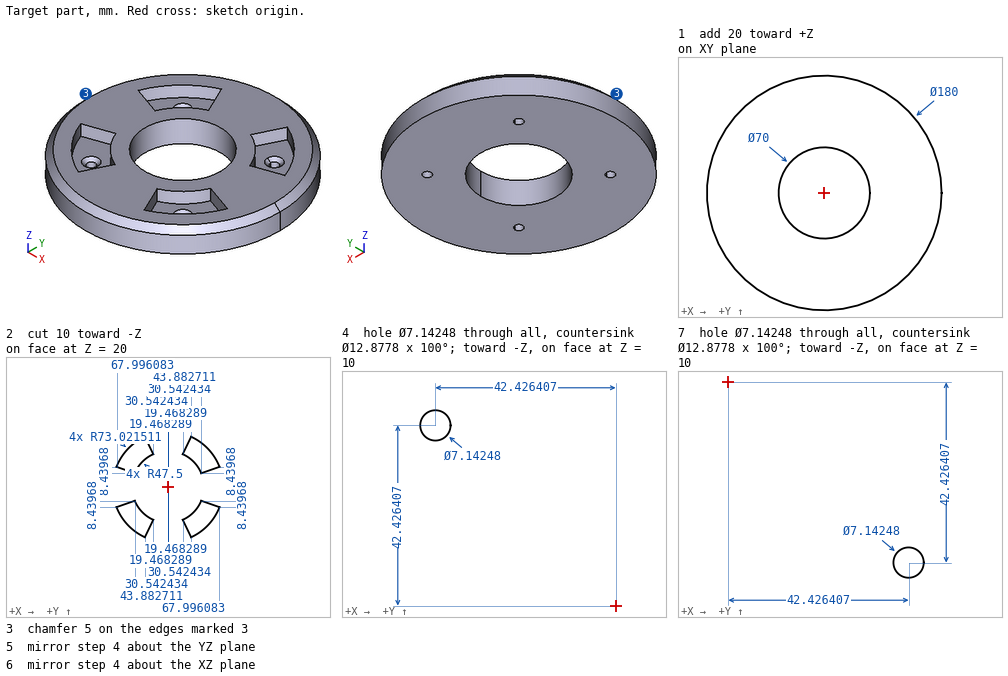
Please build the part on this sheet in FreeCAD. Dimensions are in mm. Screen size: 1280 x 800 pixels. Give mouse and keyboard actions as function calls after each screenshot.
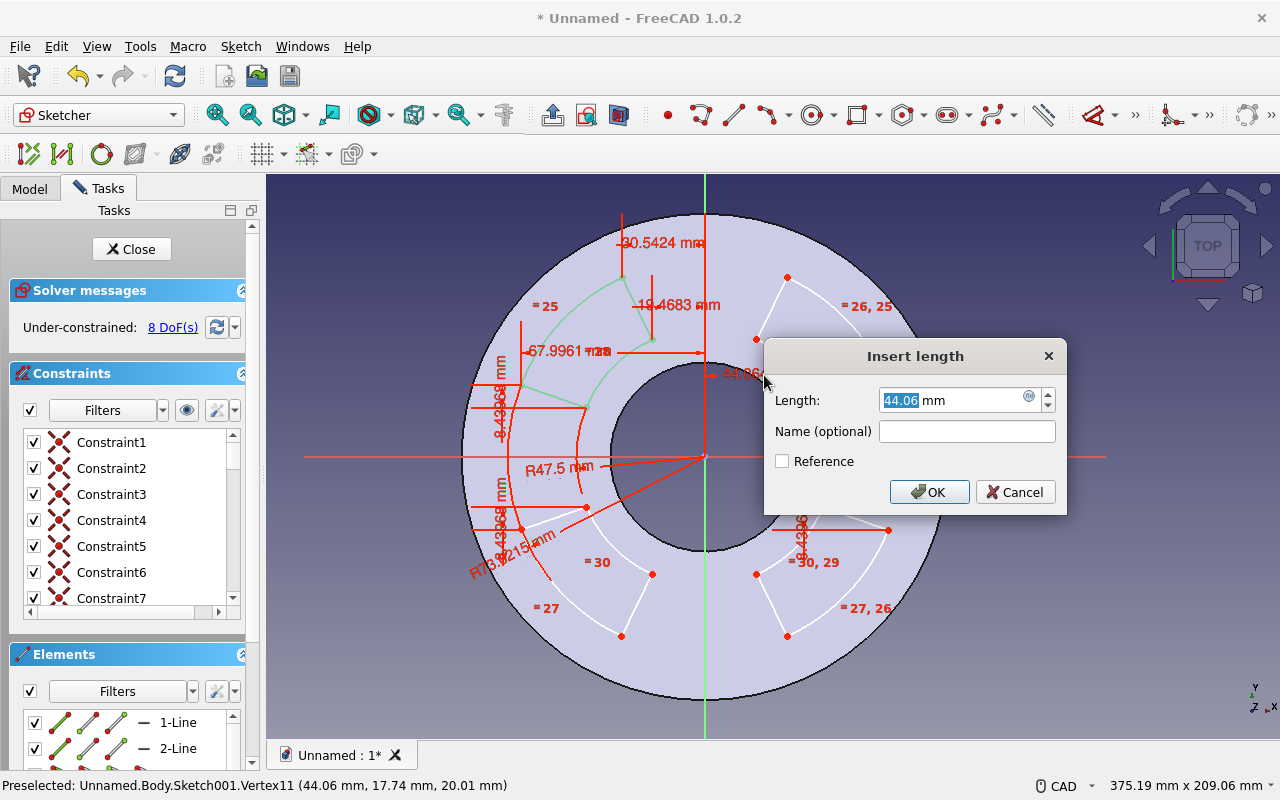
text(43.882711)
key(Return)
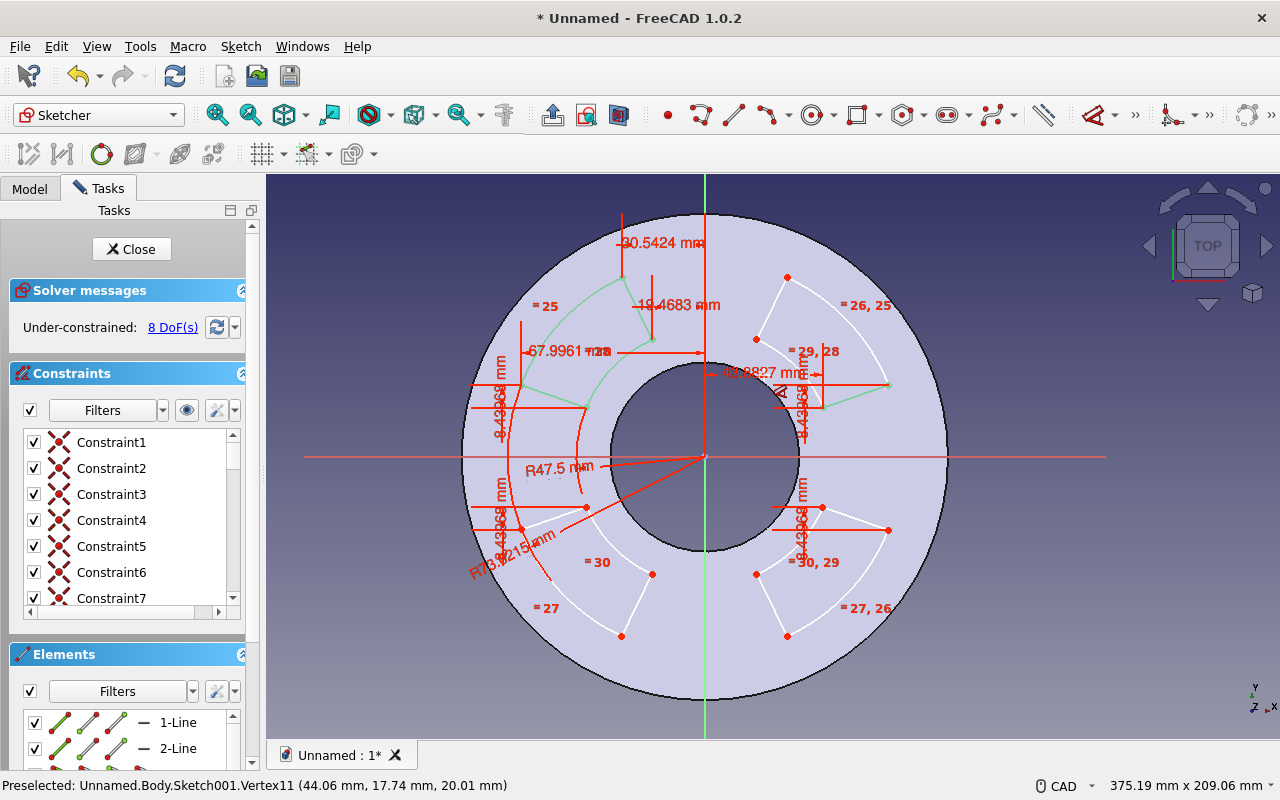
click(787, 278)
click(746, 244)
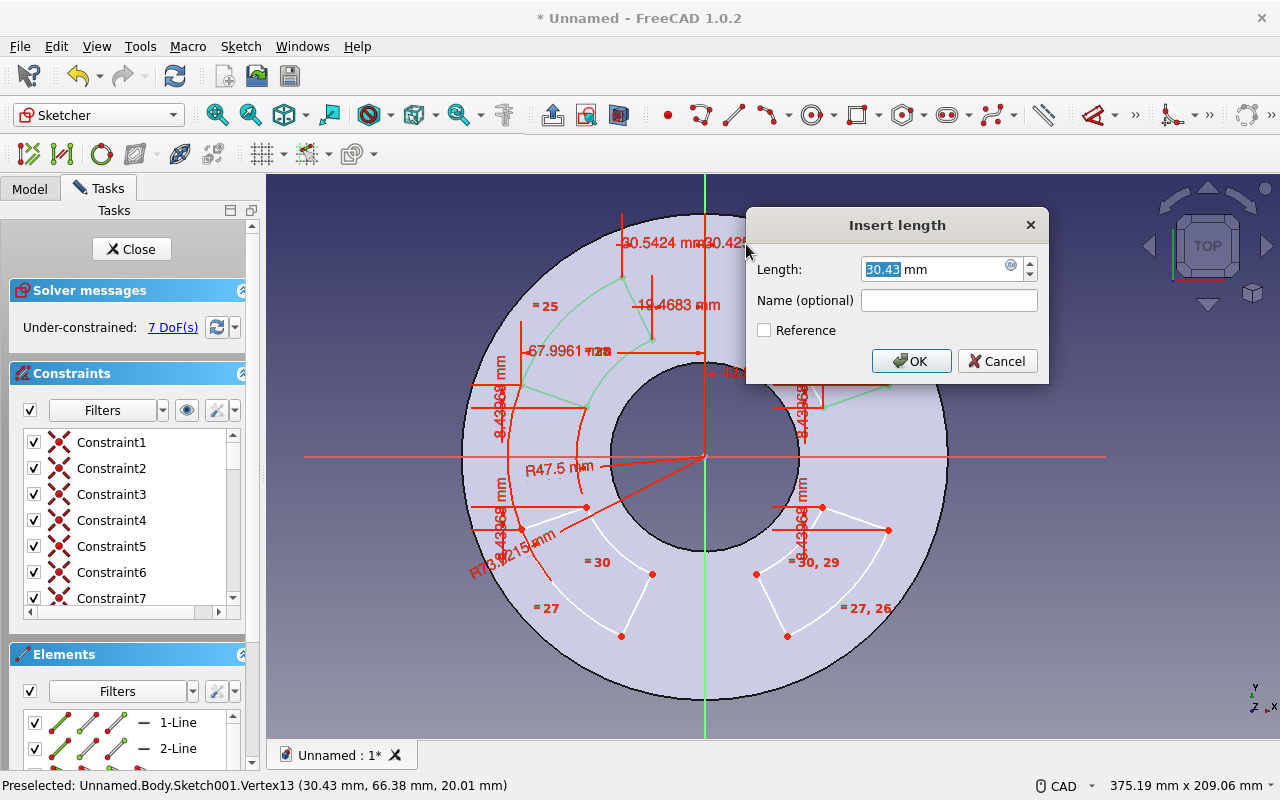
text(30.542434)
key(Return)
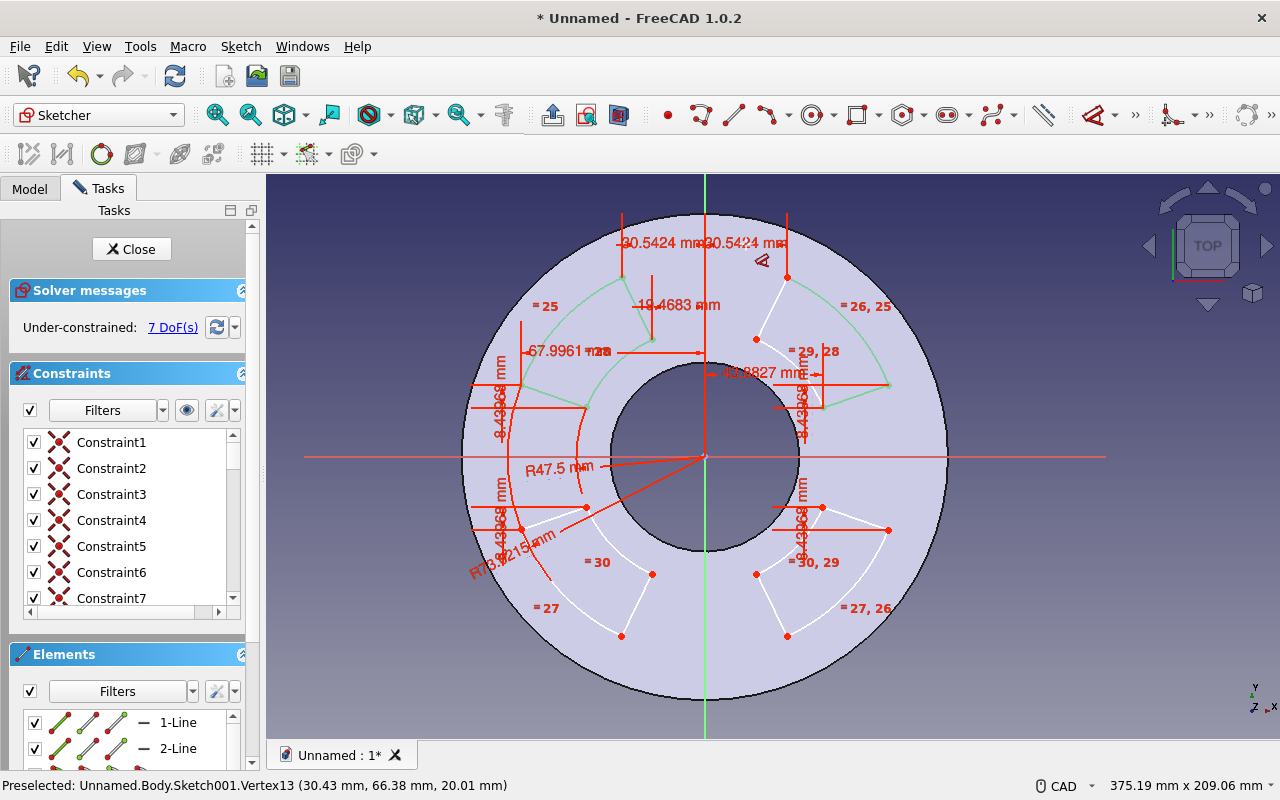
click(757, 340)
click(749, 306)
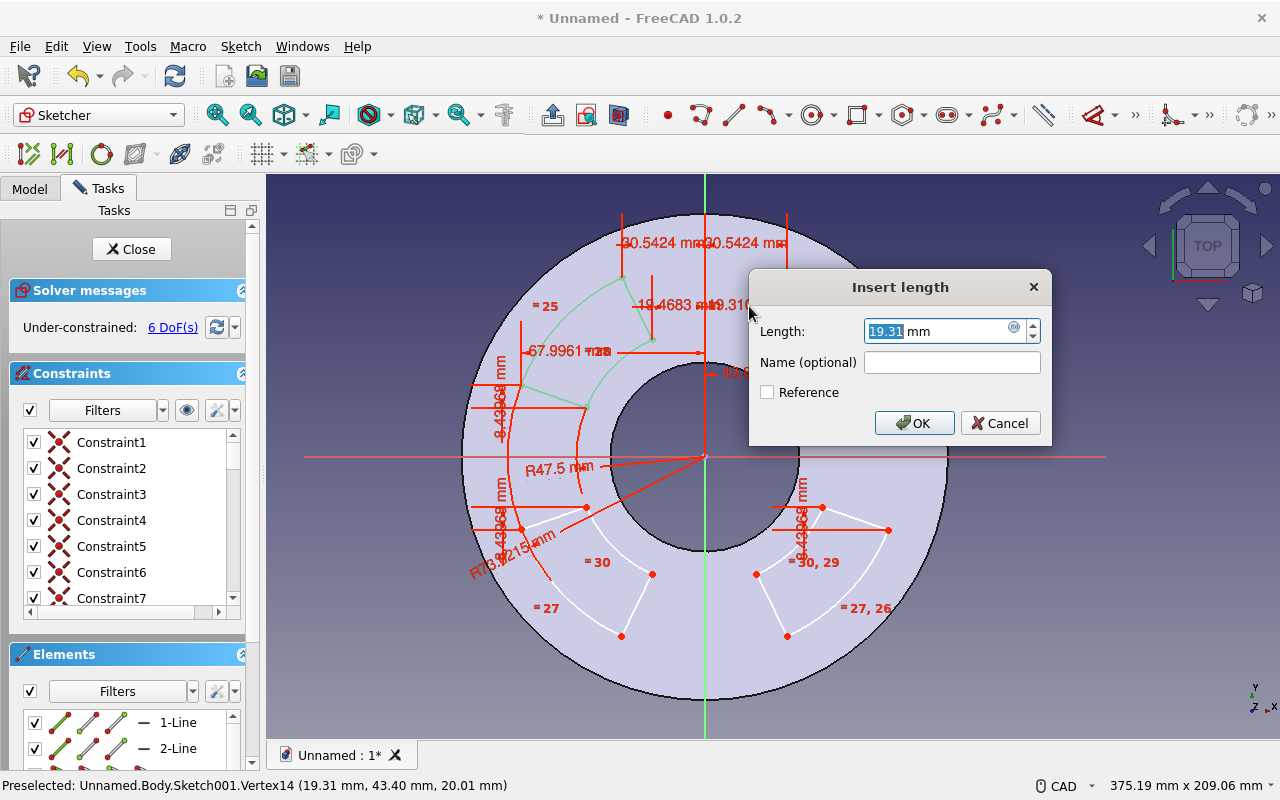
text(19.468289)
key(Return)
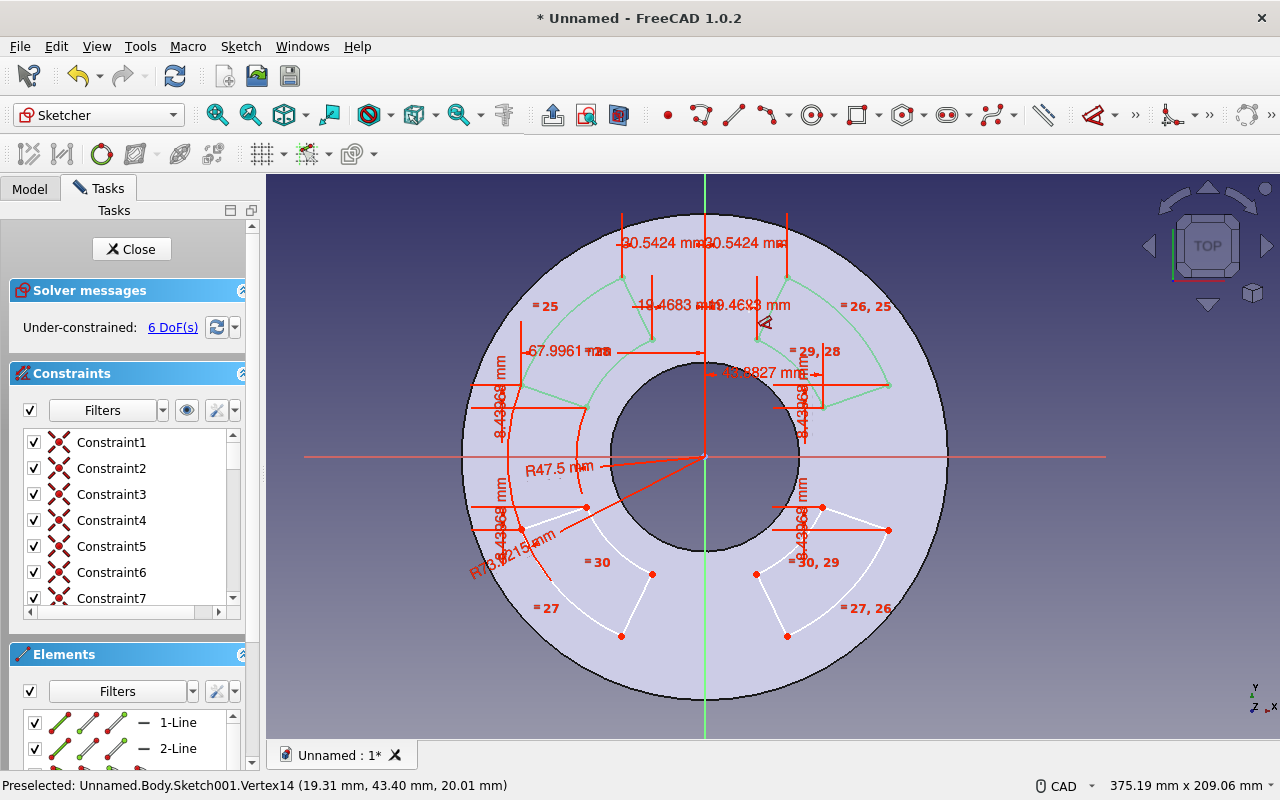
click(757, 574)
click(731, 608)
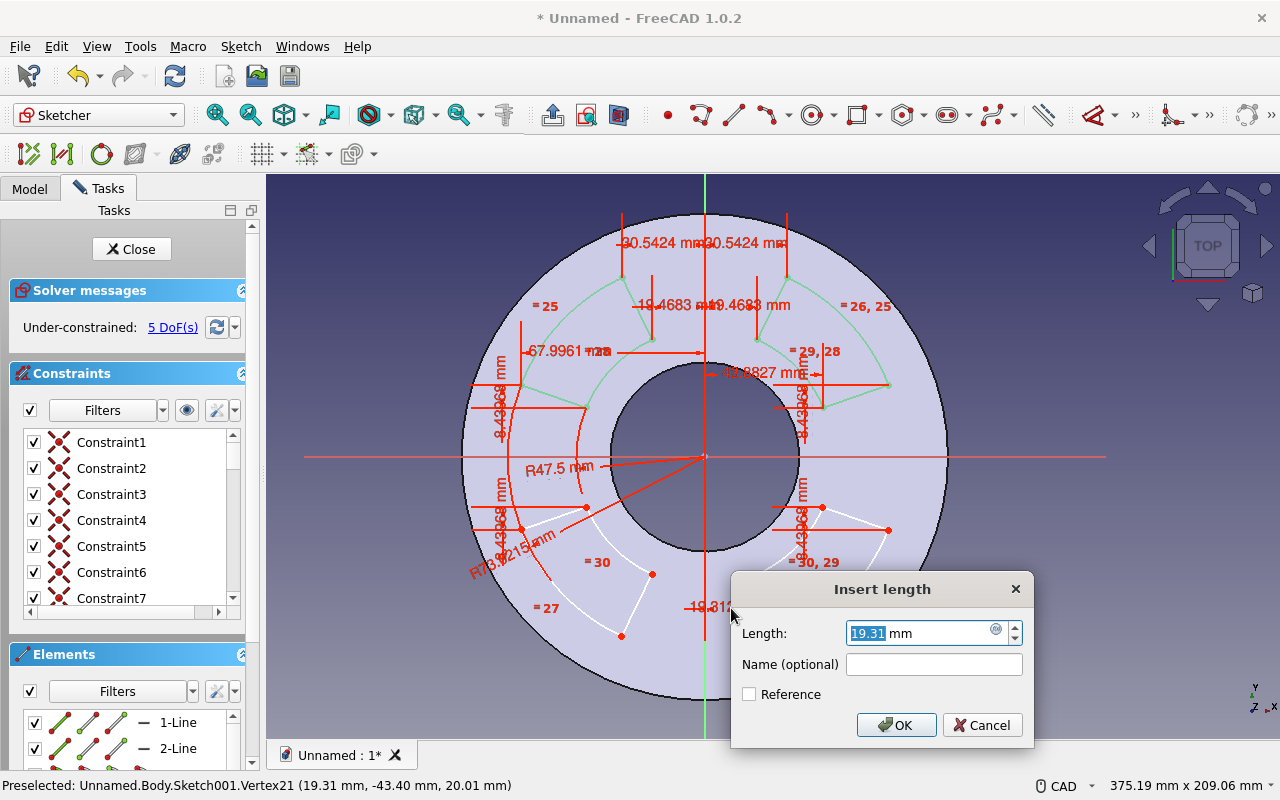
text(19.468289)
key(Return)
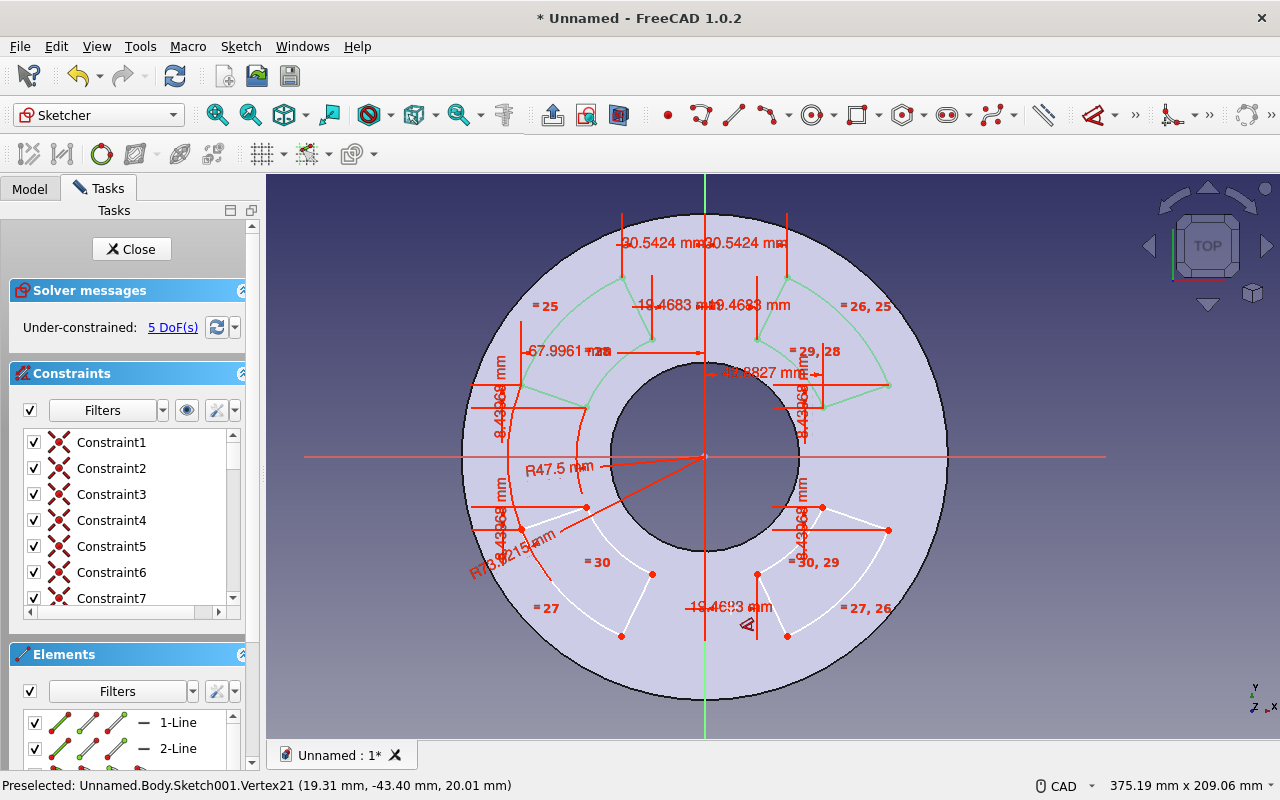
click(787, 636)
click(746, 670)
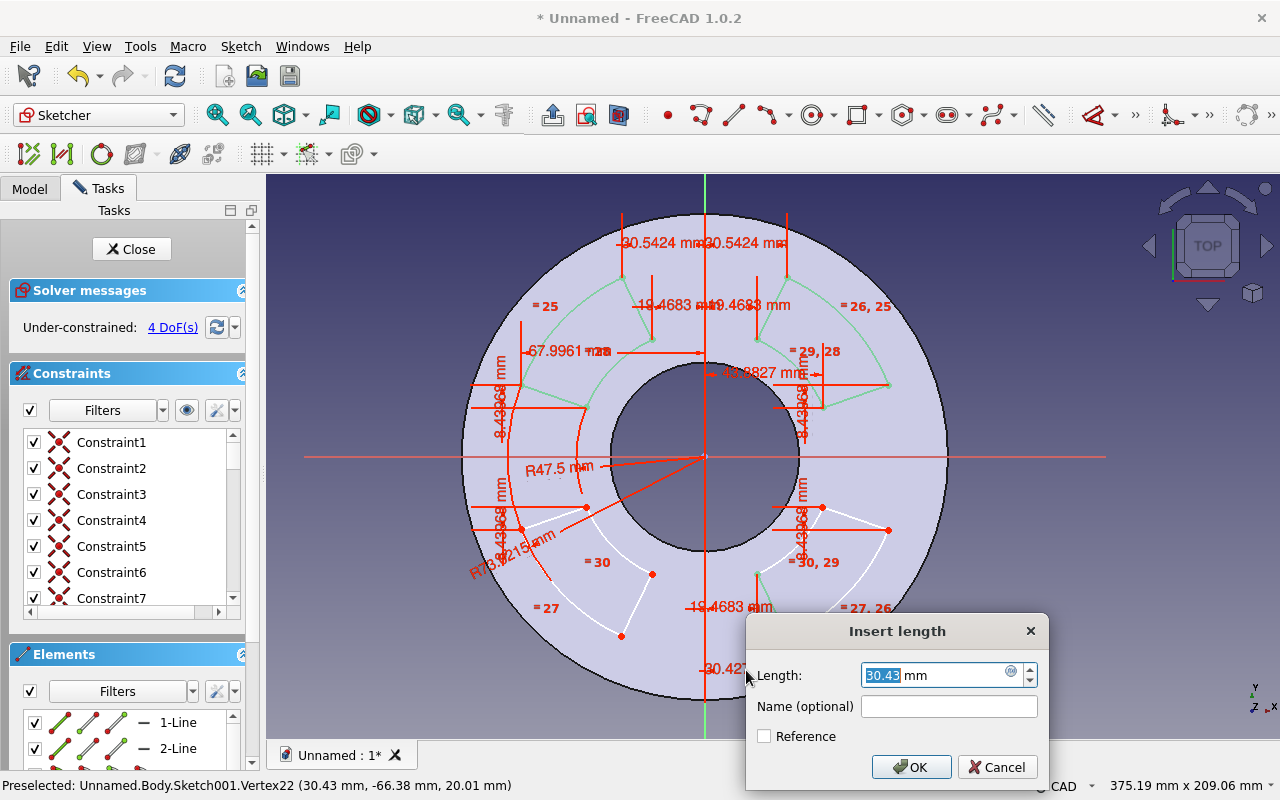
text(30.542434)
key(Return)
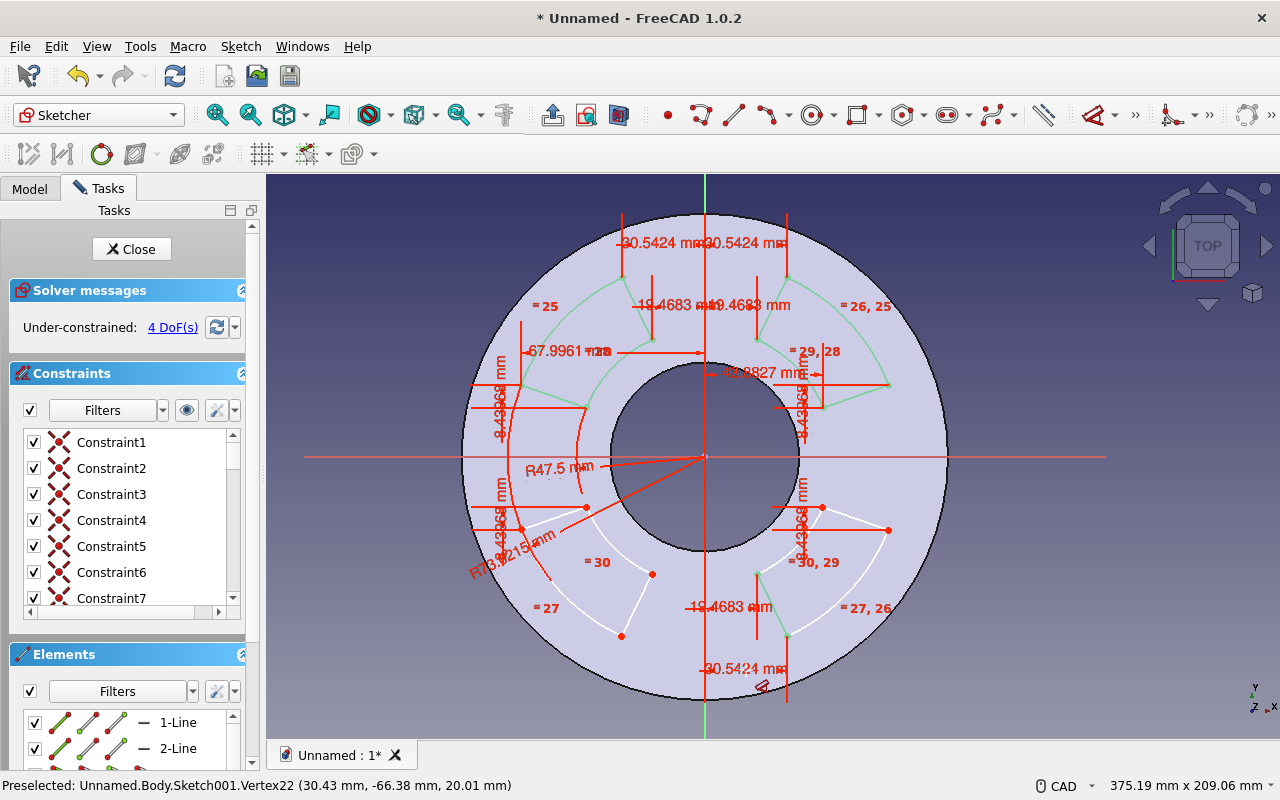
click(888, 530)
click(839, 564)